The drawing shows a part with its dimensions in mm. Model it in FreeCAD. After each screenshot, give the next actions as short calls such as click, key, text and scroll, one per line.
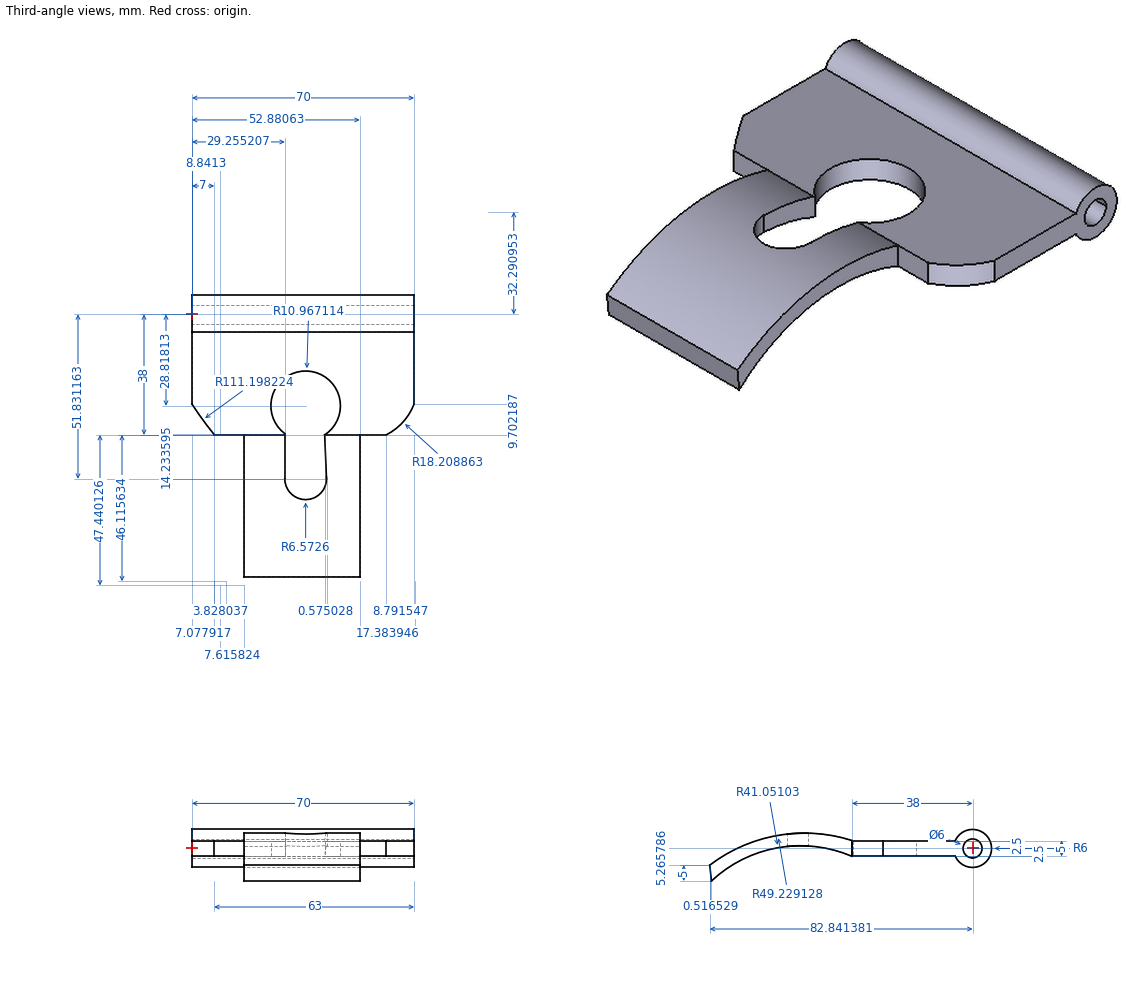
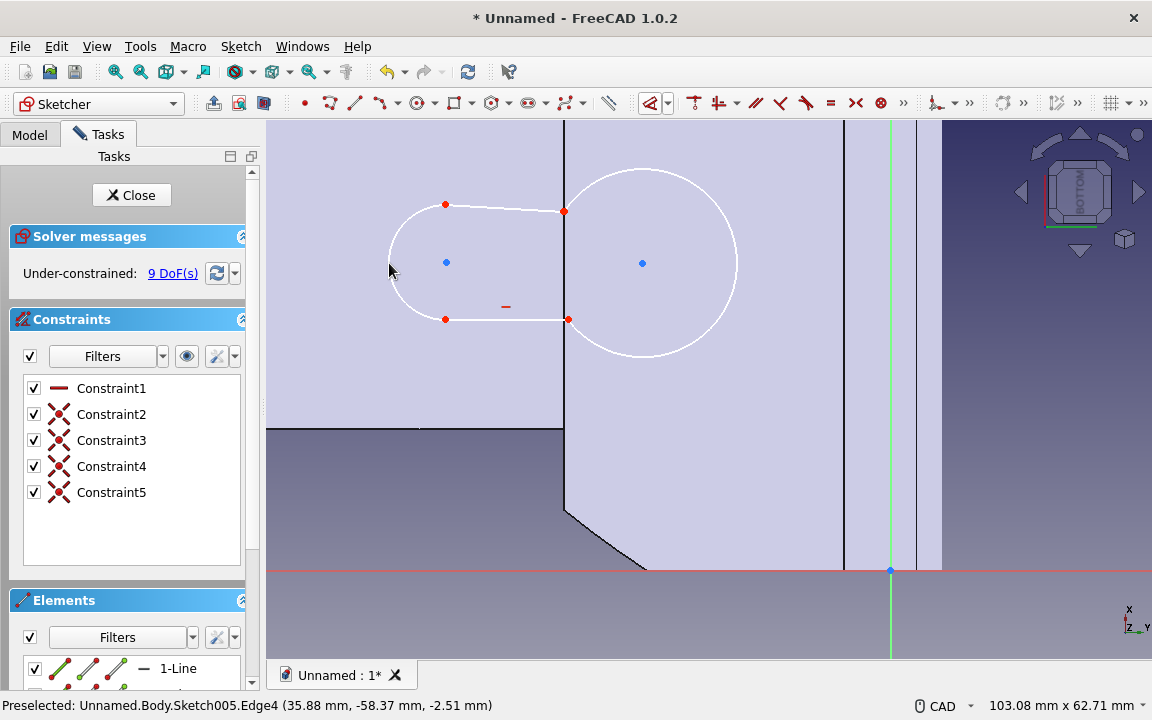
click(482, 320)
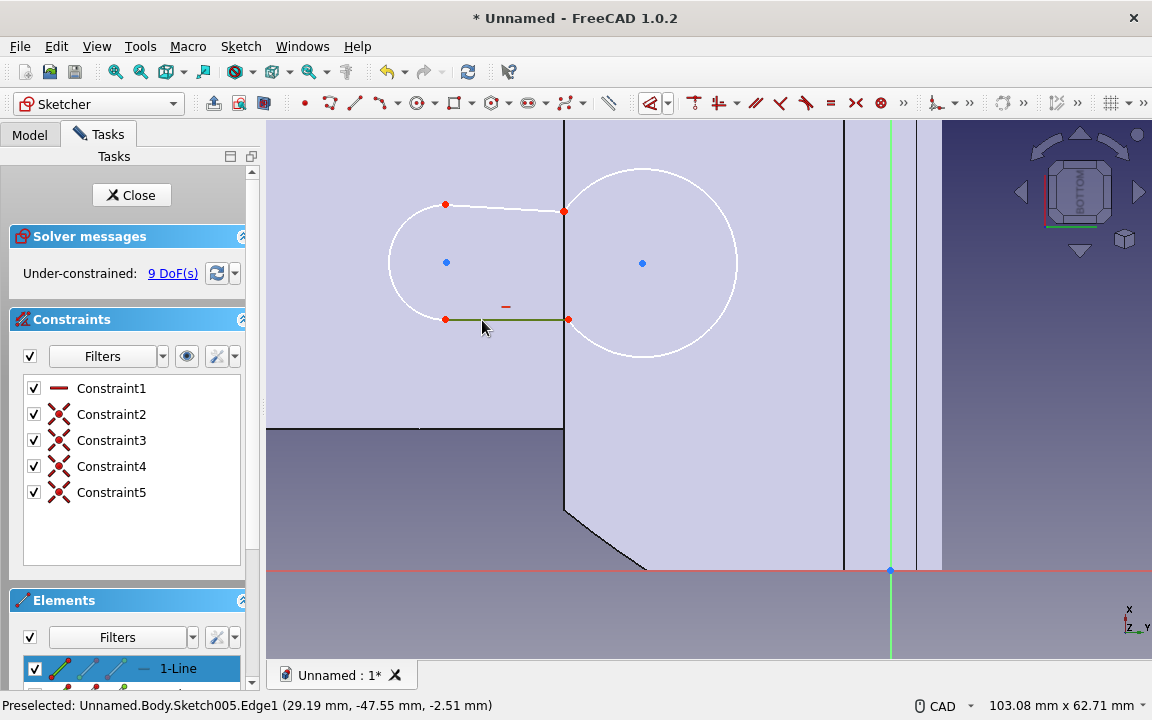
click(400, 229)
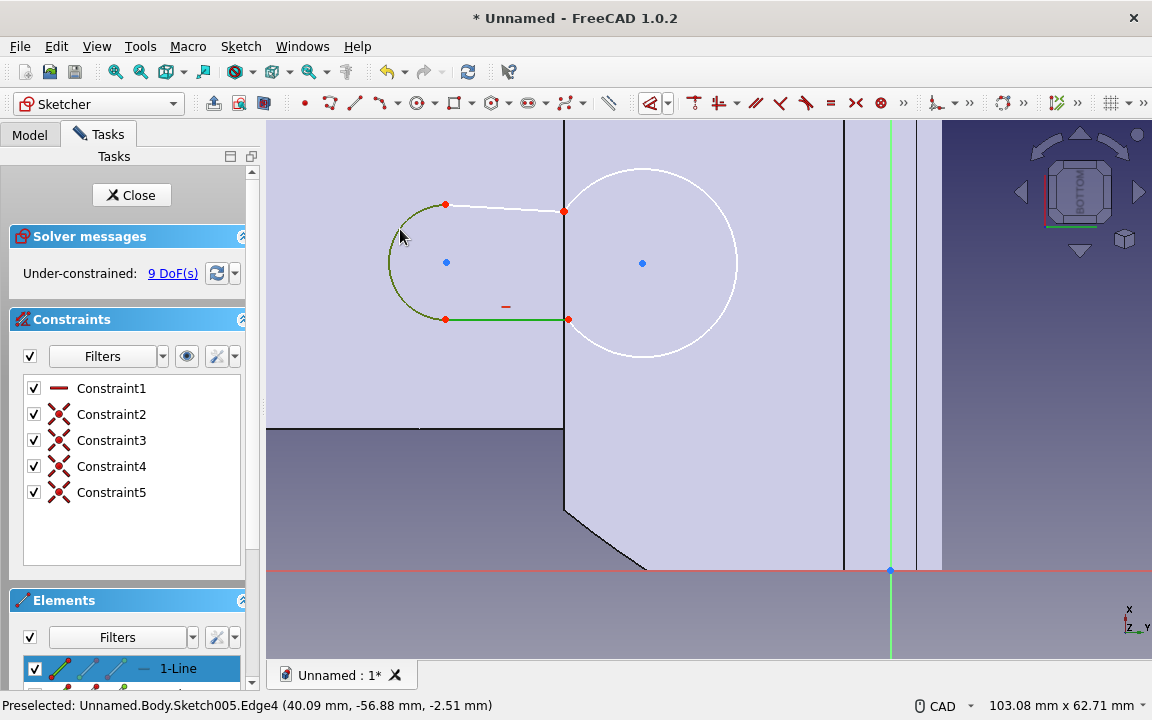
click(806, 104)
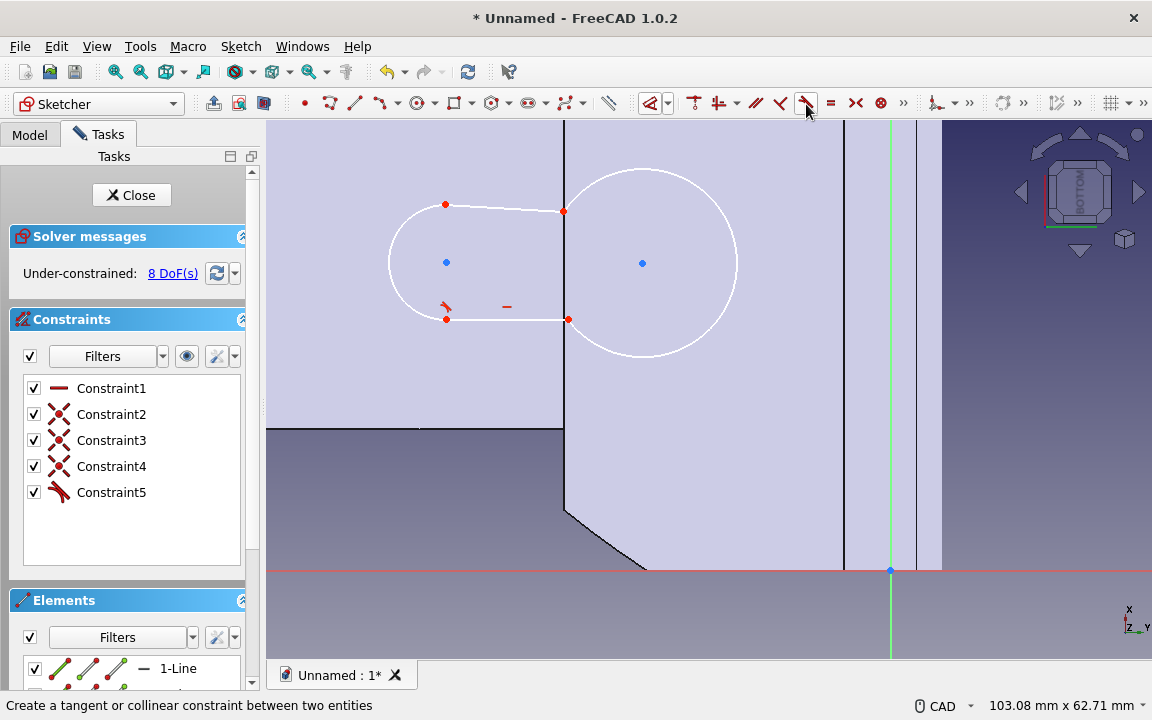
click(696, 341)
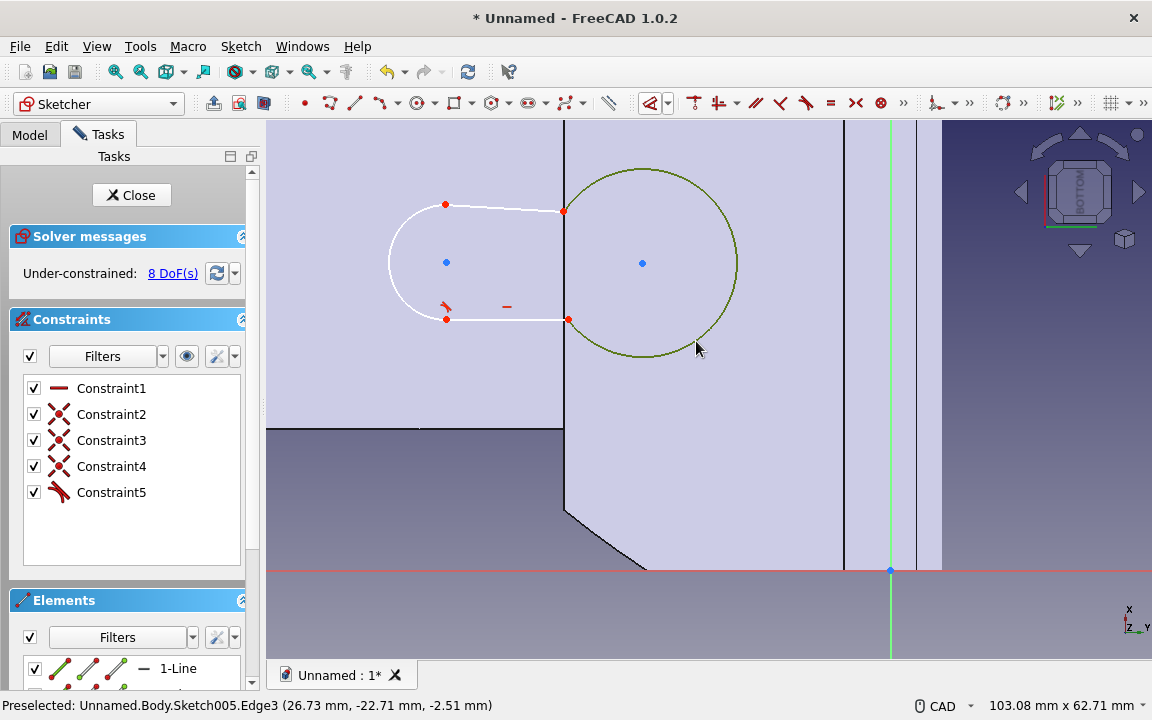
click(668, 104)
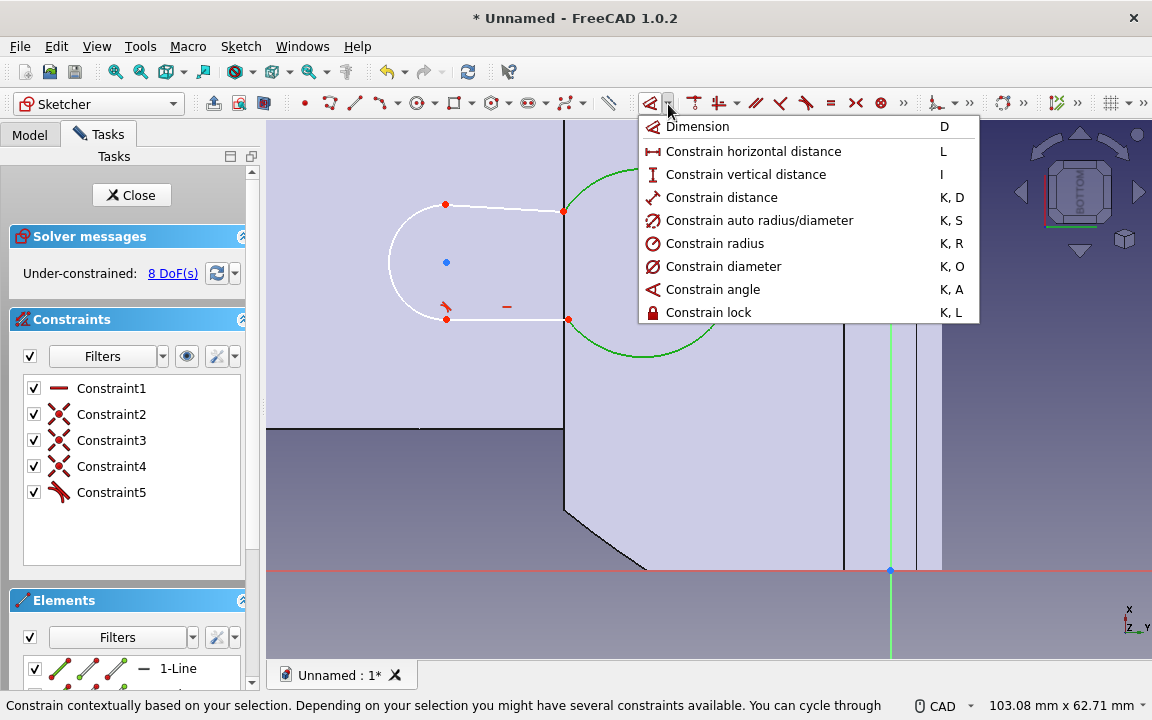
click(809, 244)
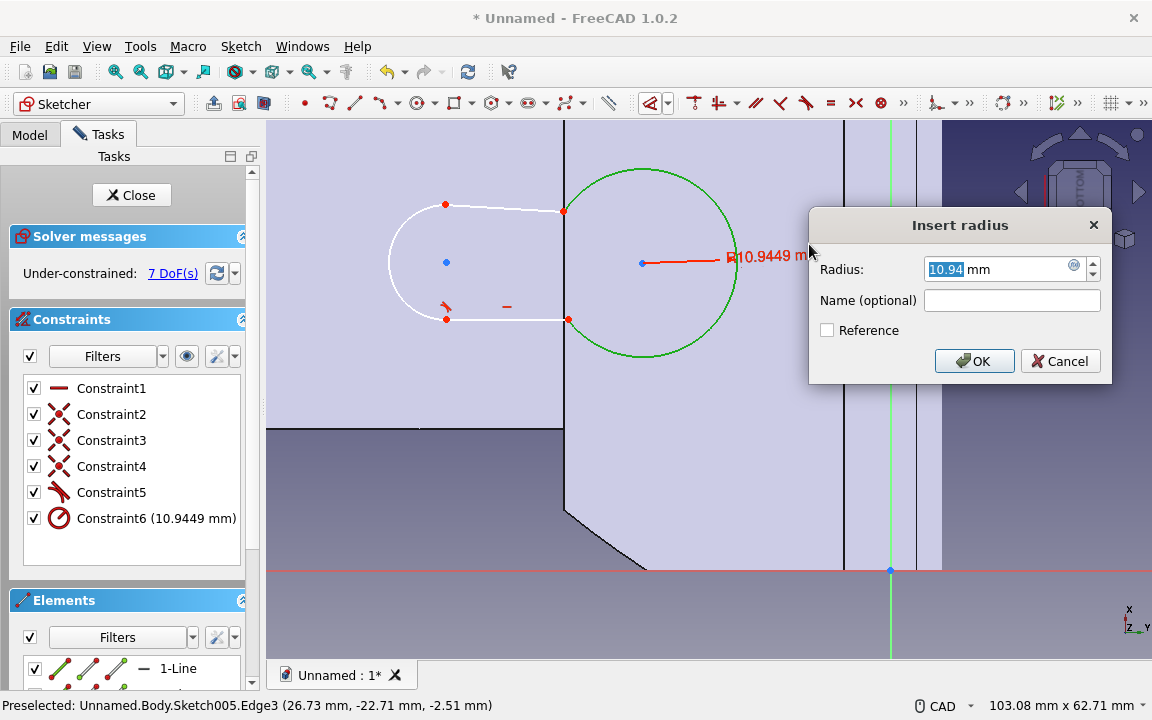
text(10.967114)
key(Return)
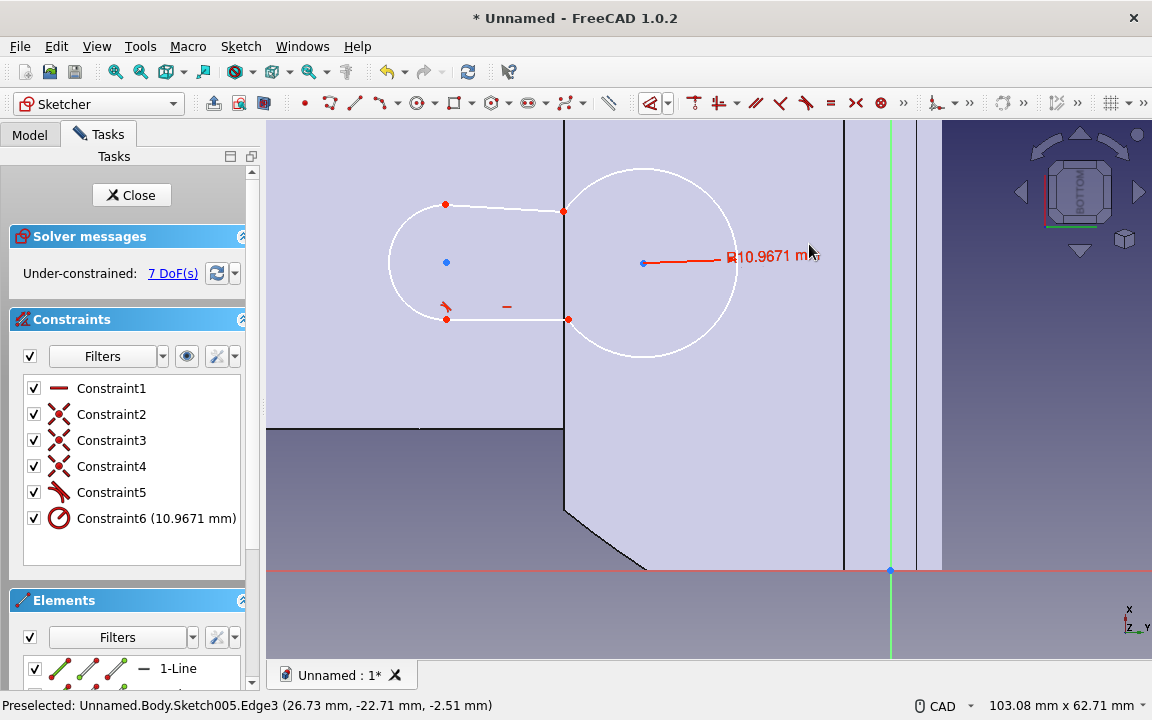
click(399, 230)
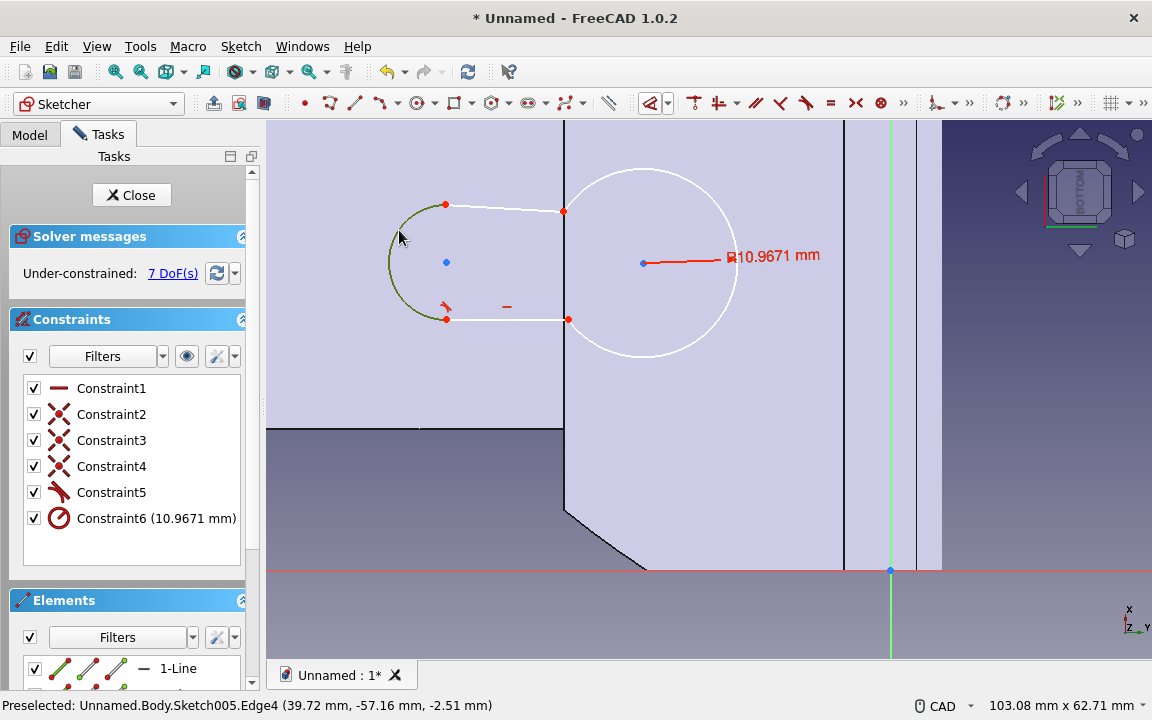
click(668, 104)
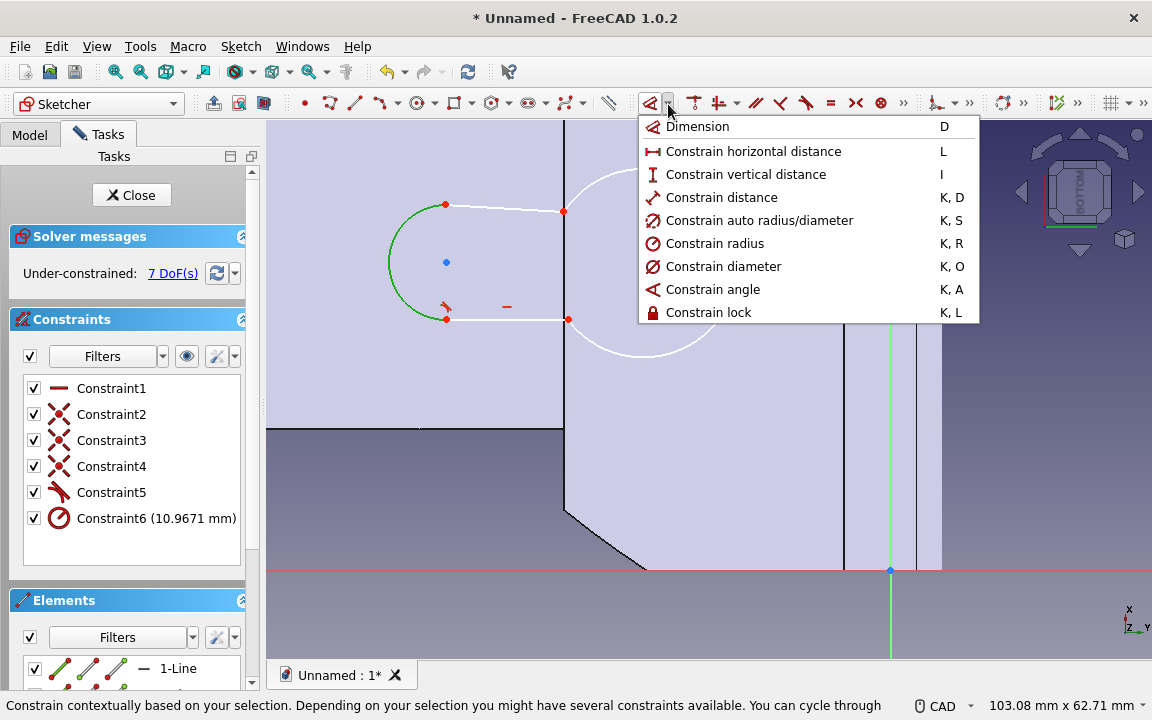
click(809, 244)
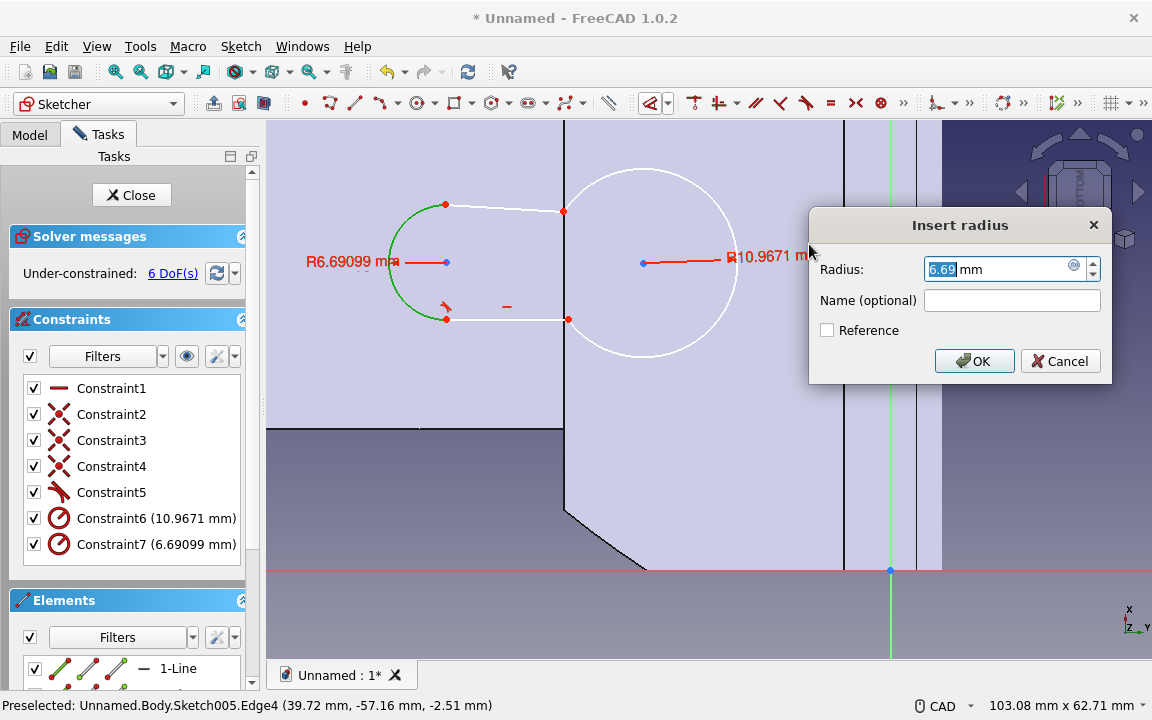
text(6.5726)
key(Return)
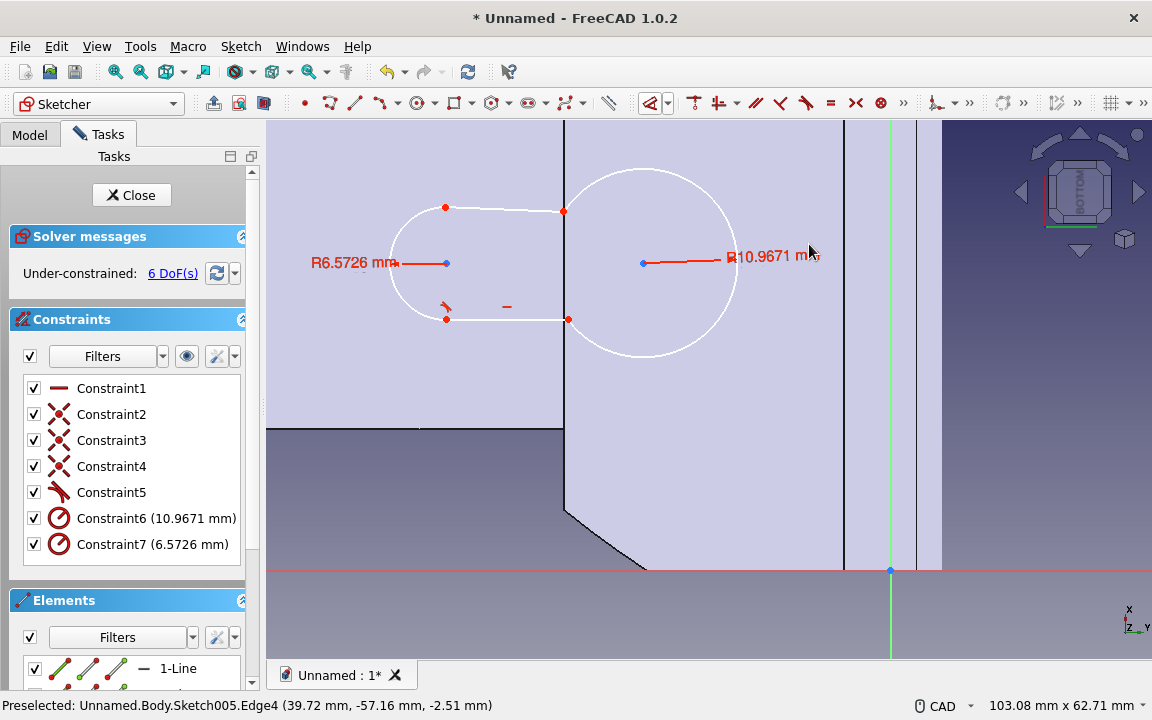
click(564, 212)